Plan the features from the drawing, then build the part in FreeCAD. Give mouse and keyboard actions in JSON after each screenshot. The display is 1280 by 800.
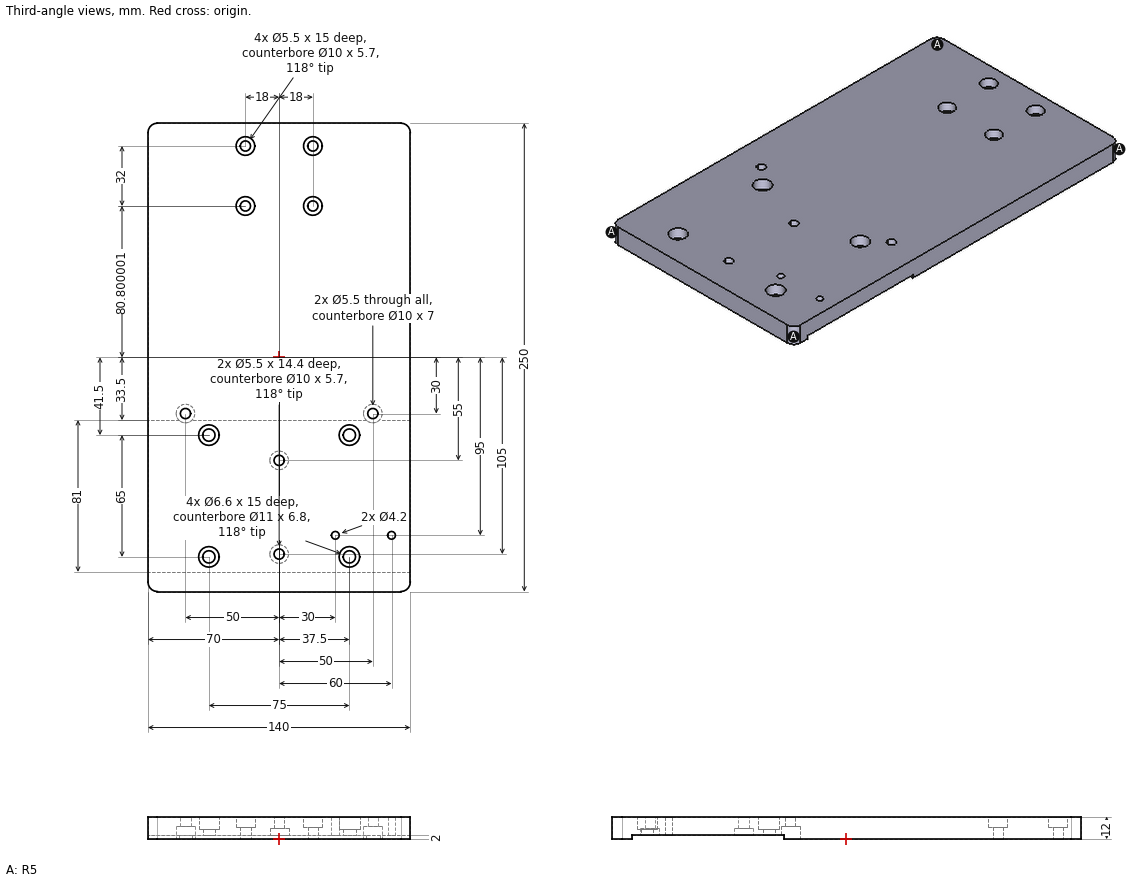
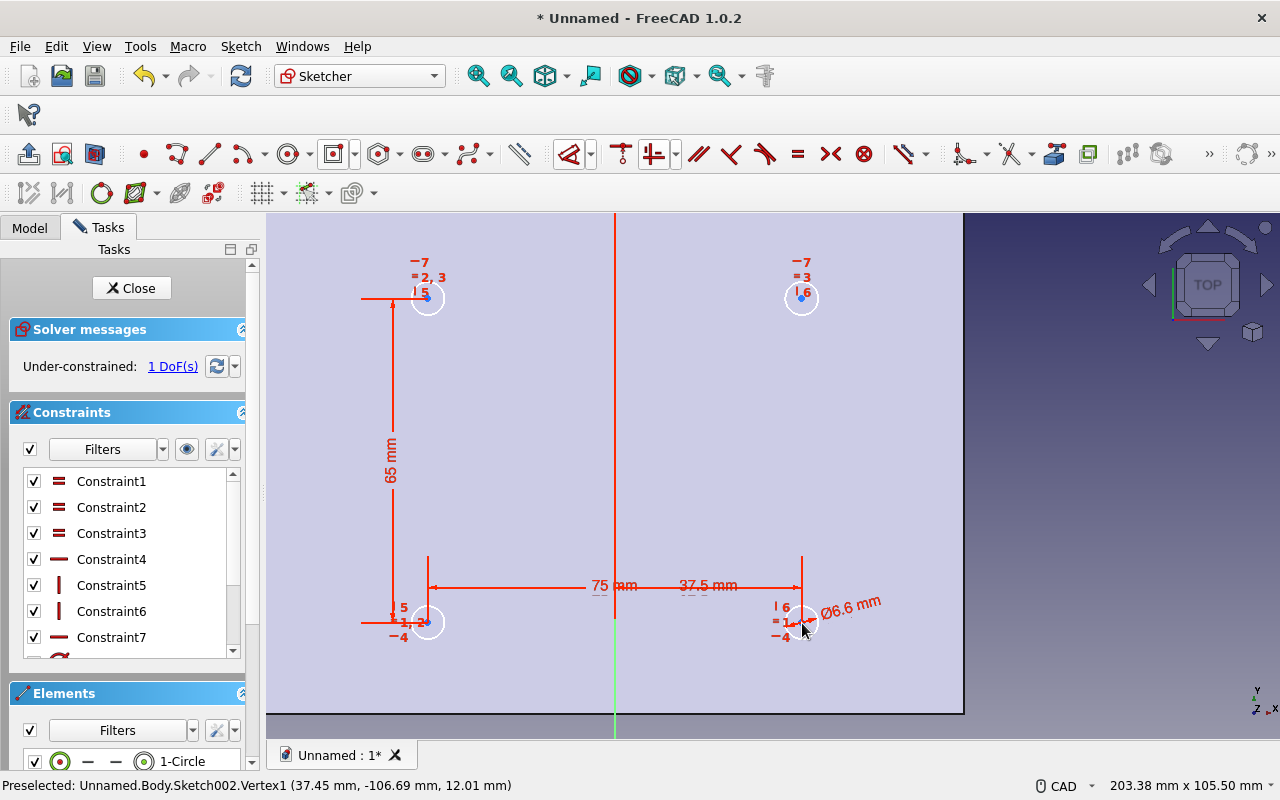
{"action": "left_click", "coordinate": [428, 299]}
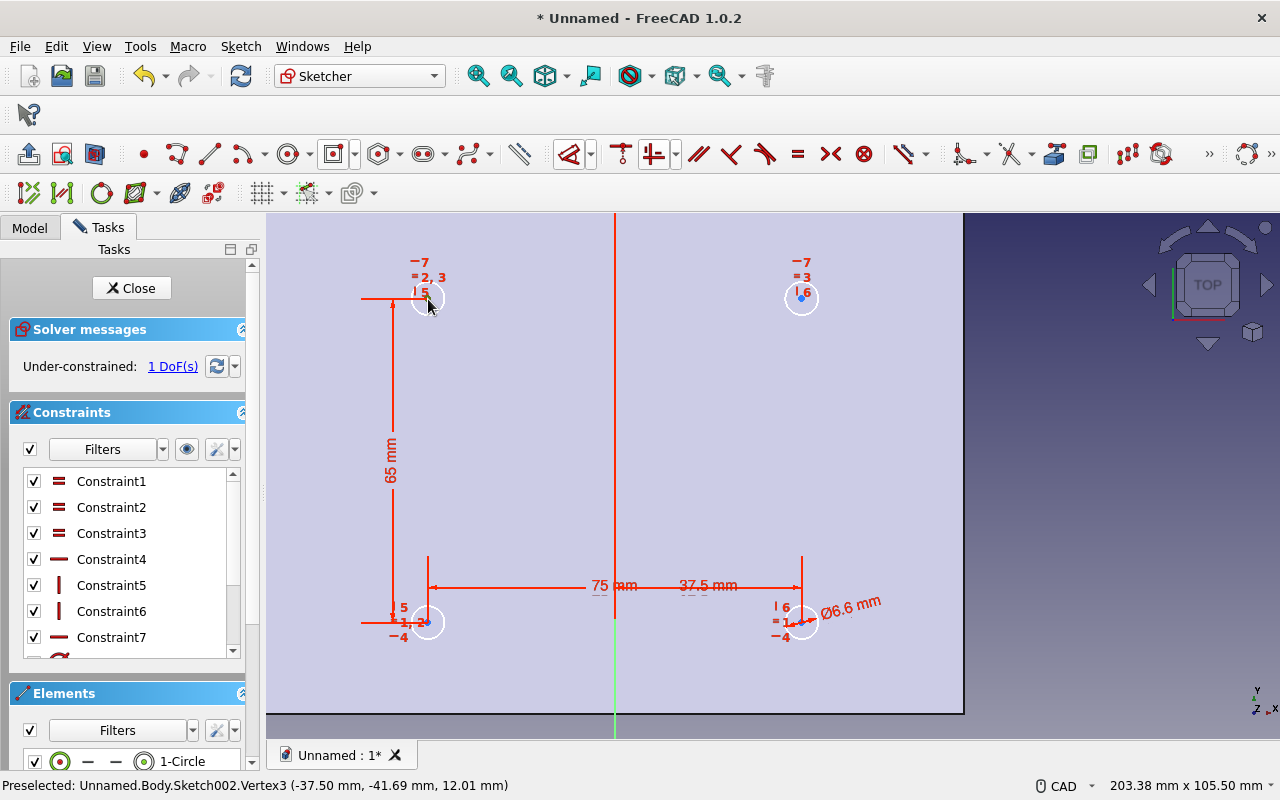
{"action": "left_click", "coordinate": [590, 154]}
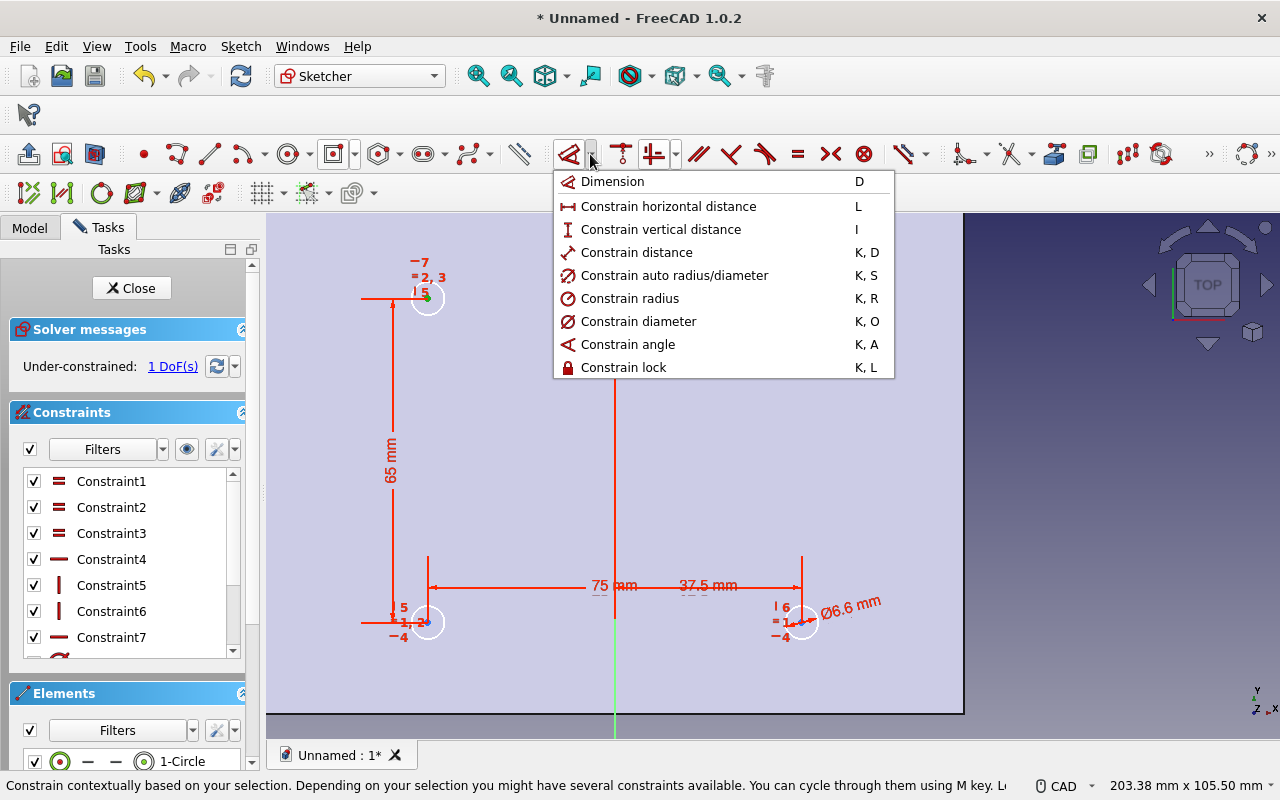
{"action": "left_click", "coordinate": [724, 230]}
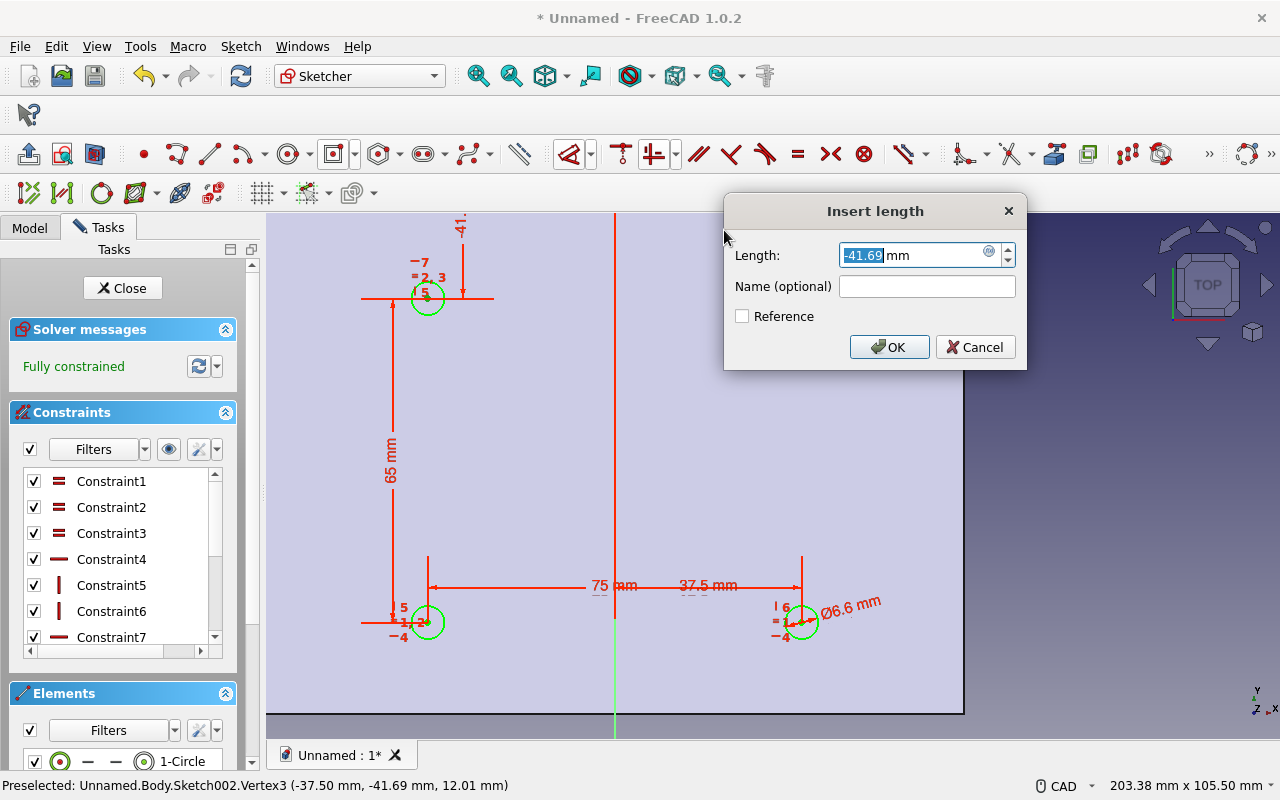
{"action": "type", "text": "-41.5"}
{"action": "key", "text": "Return"}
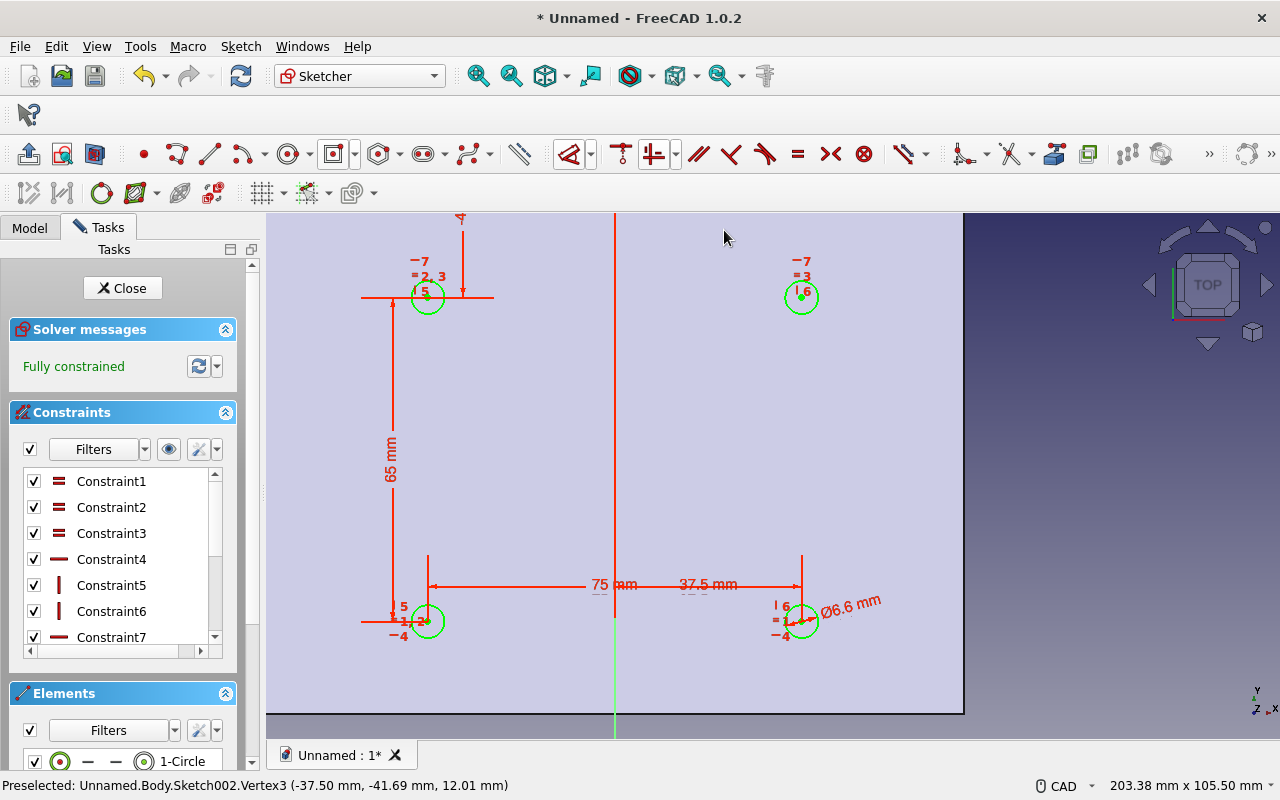
{"action": "left_click", "coordinate": [123, 288]}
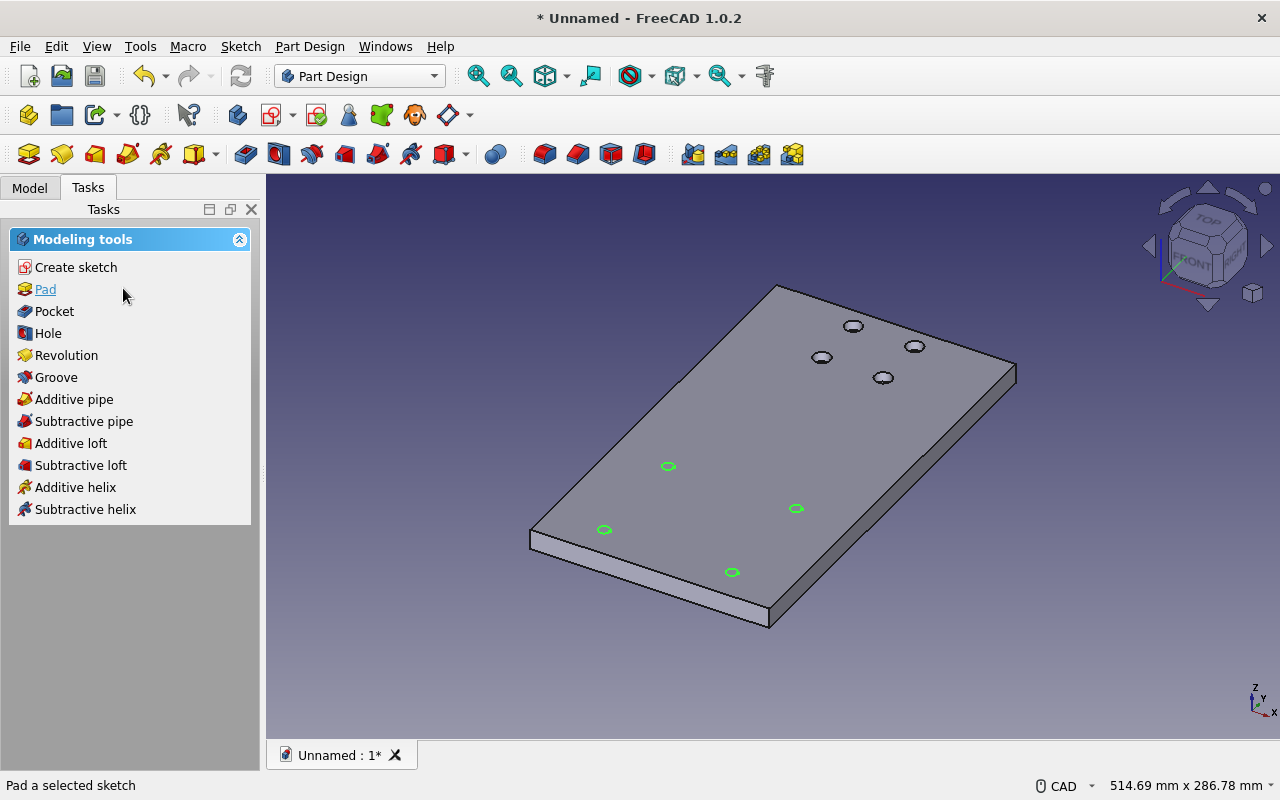
{"action": "left_click", "coordinate": [279, 154]}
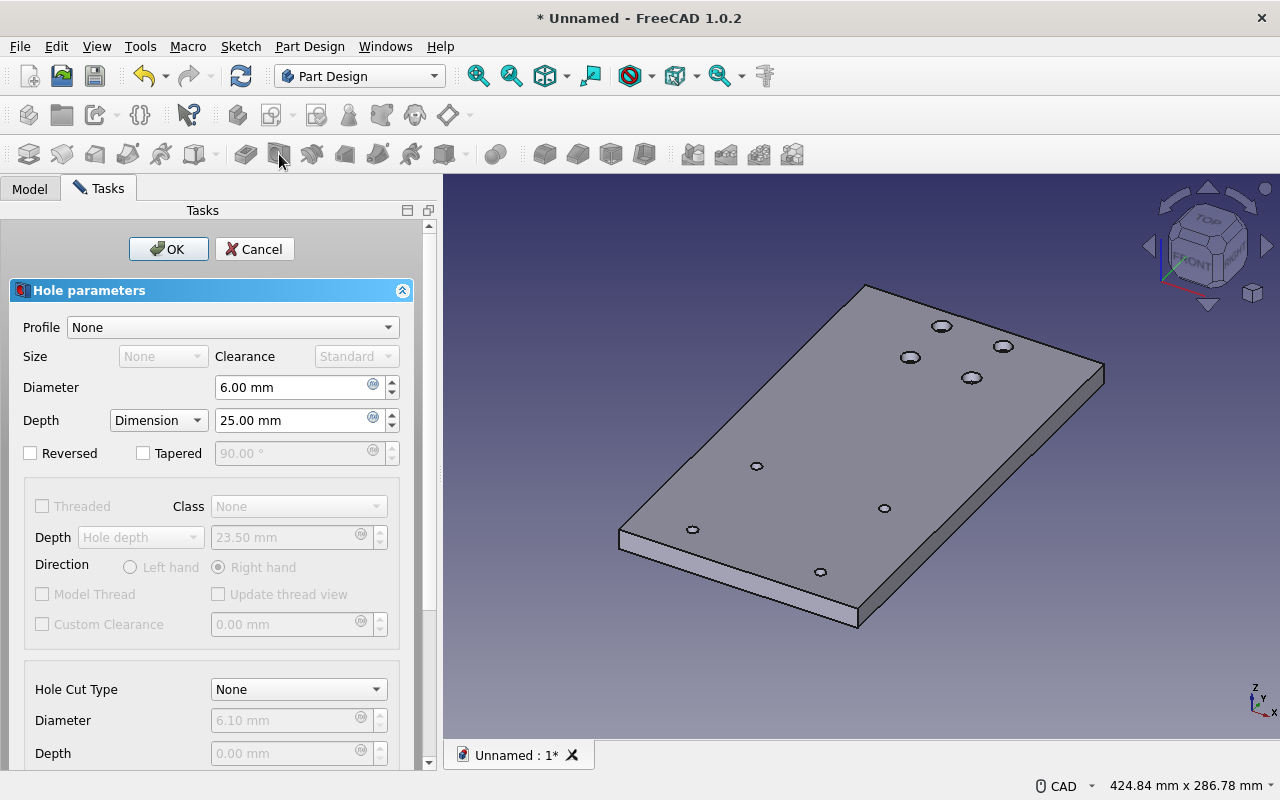
{"action": "triple_click", "coordinate": [300, 388]}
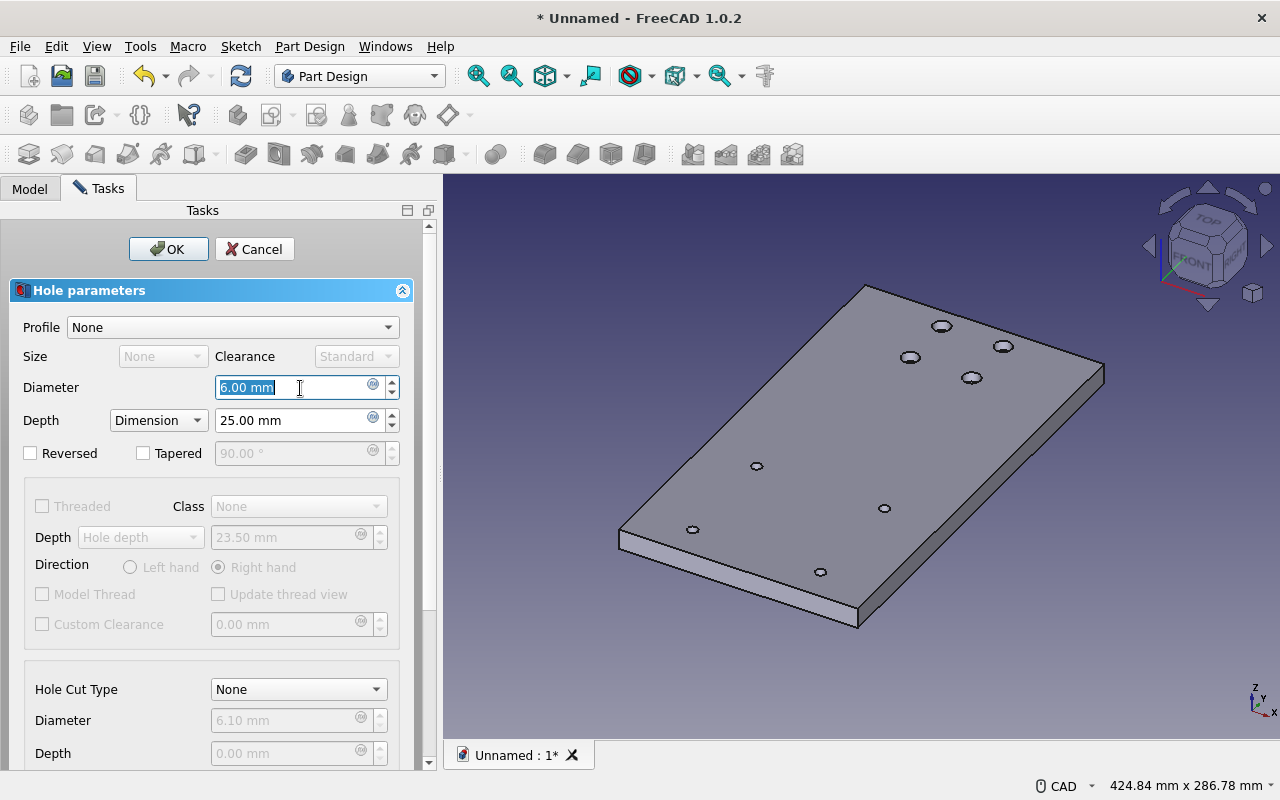
{"action": "type", "text": "6.6"}
{"action": "key", "text": "Tab"}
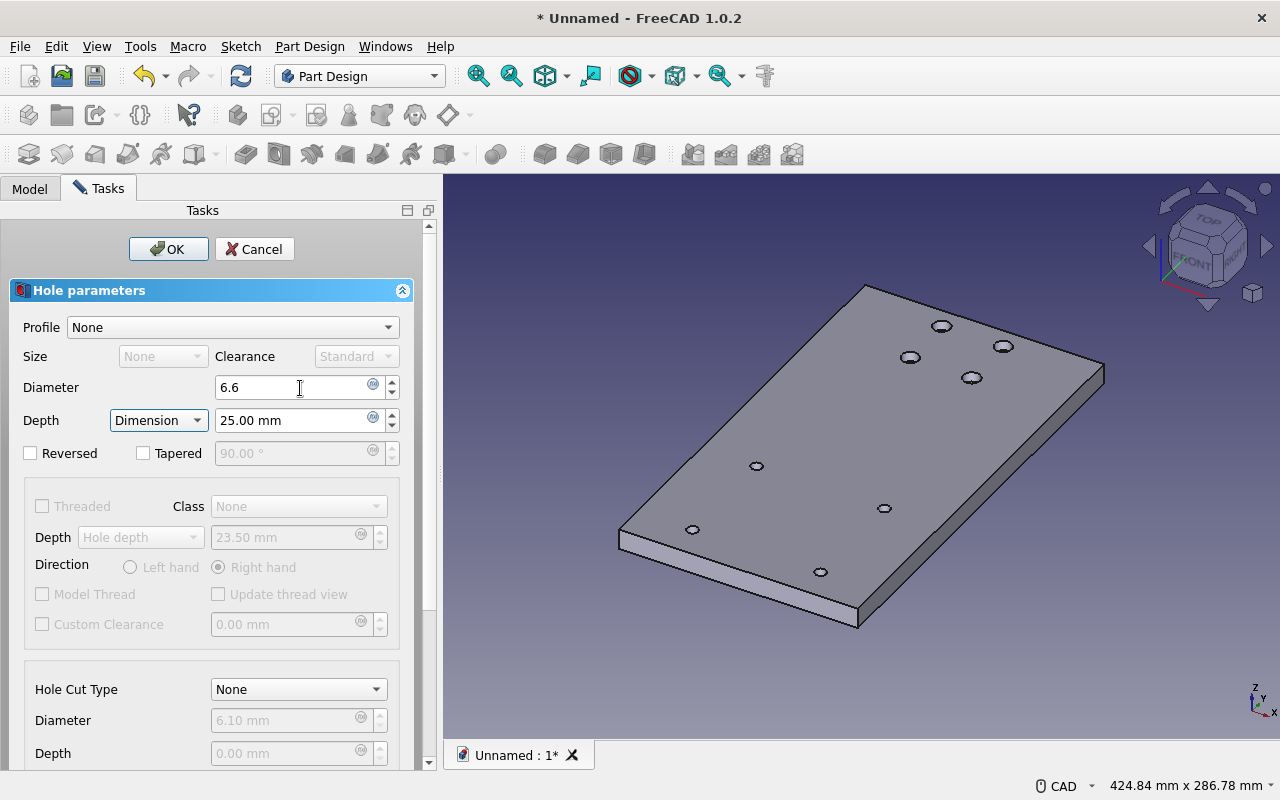
{"action": "triple_click", "coordinate": [300, 420]}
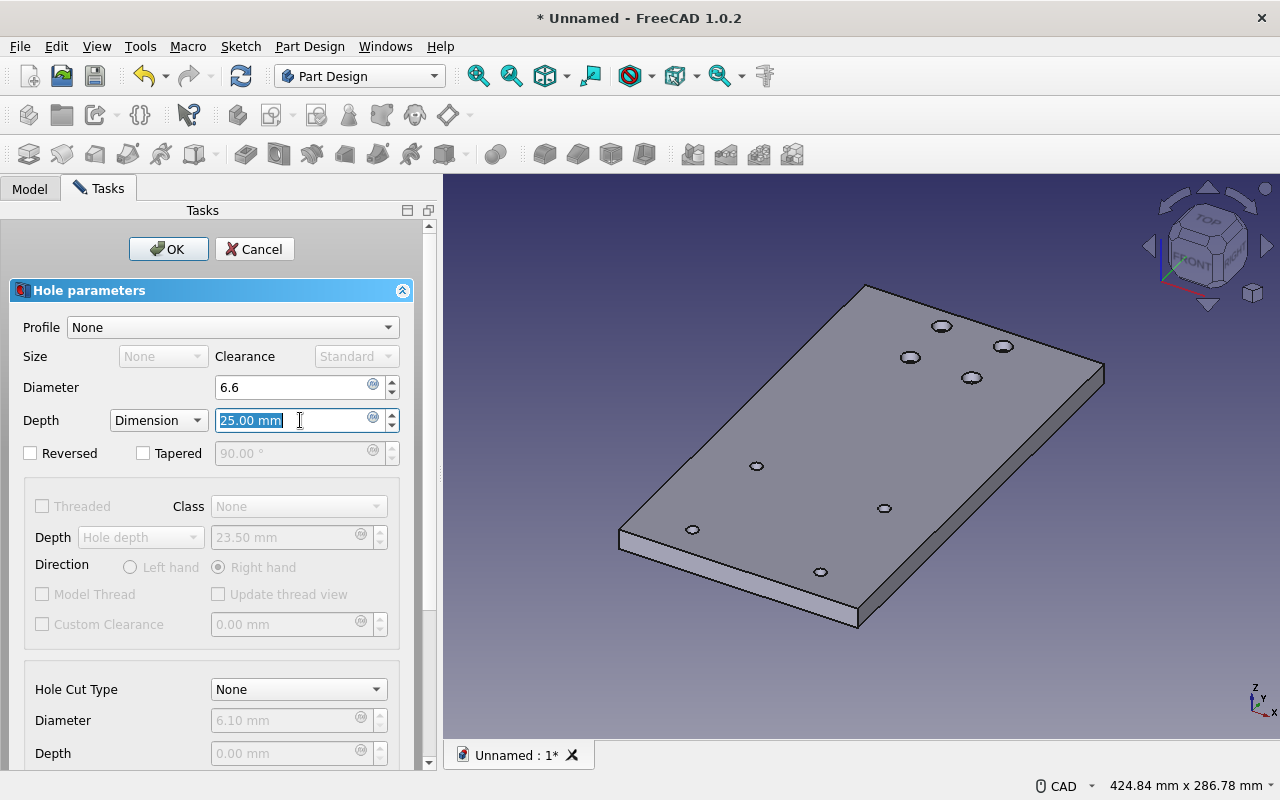
{"action": "type", "text": "15"}
{"action": "key", "text": "Tab"}